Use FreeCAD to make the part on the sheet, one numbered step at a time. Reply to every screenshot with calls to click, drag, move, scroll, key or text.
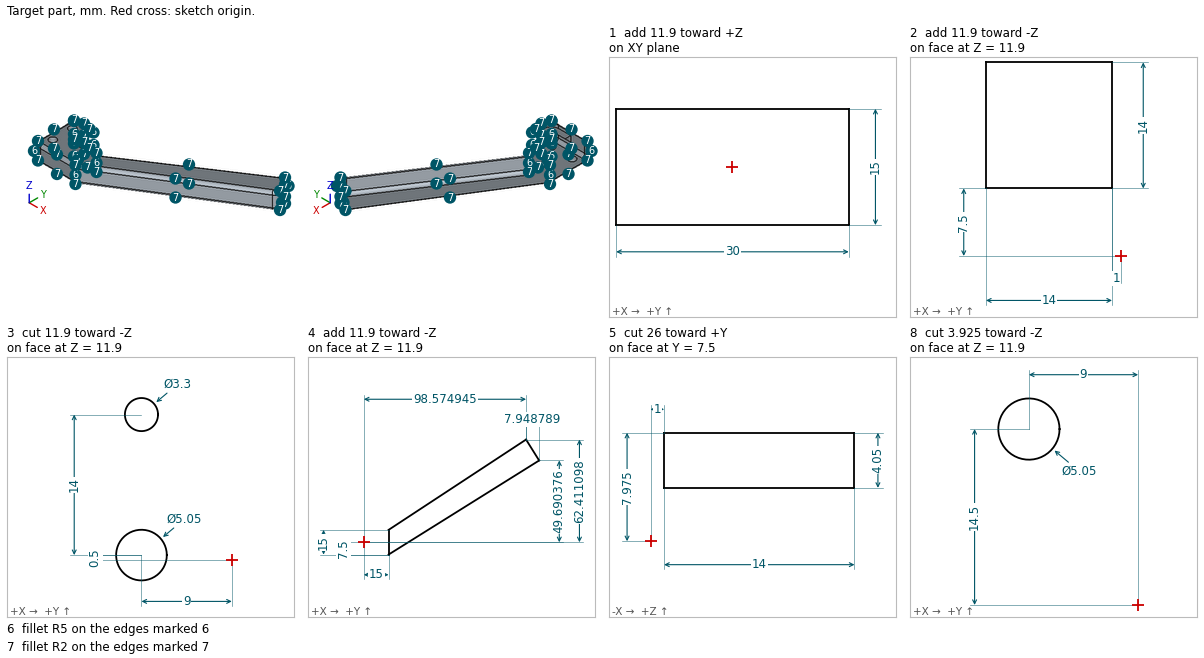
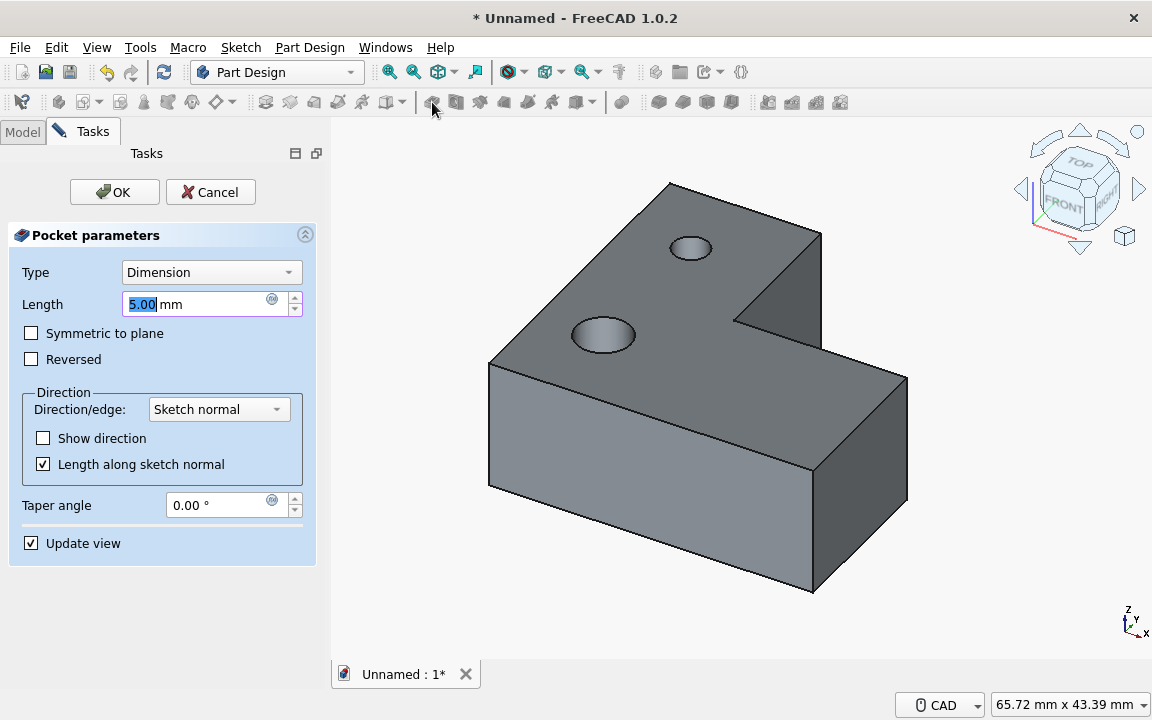
text(11.9)
key(Tab)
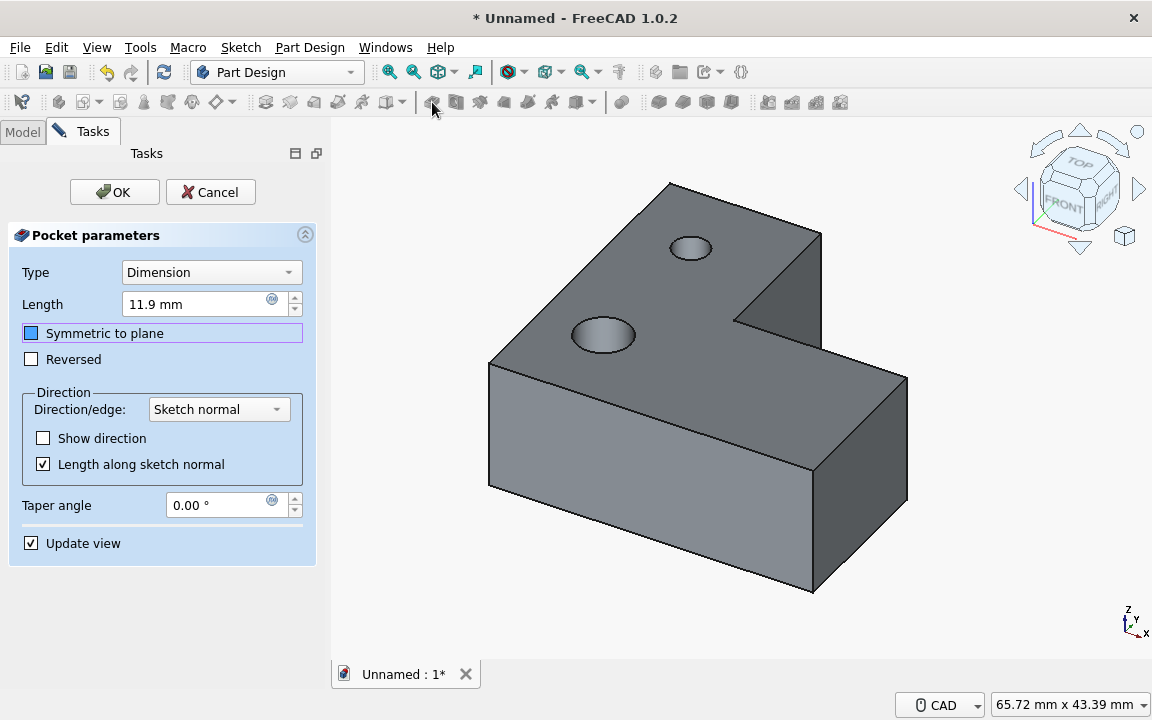
click(115, 192)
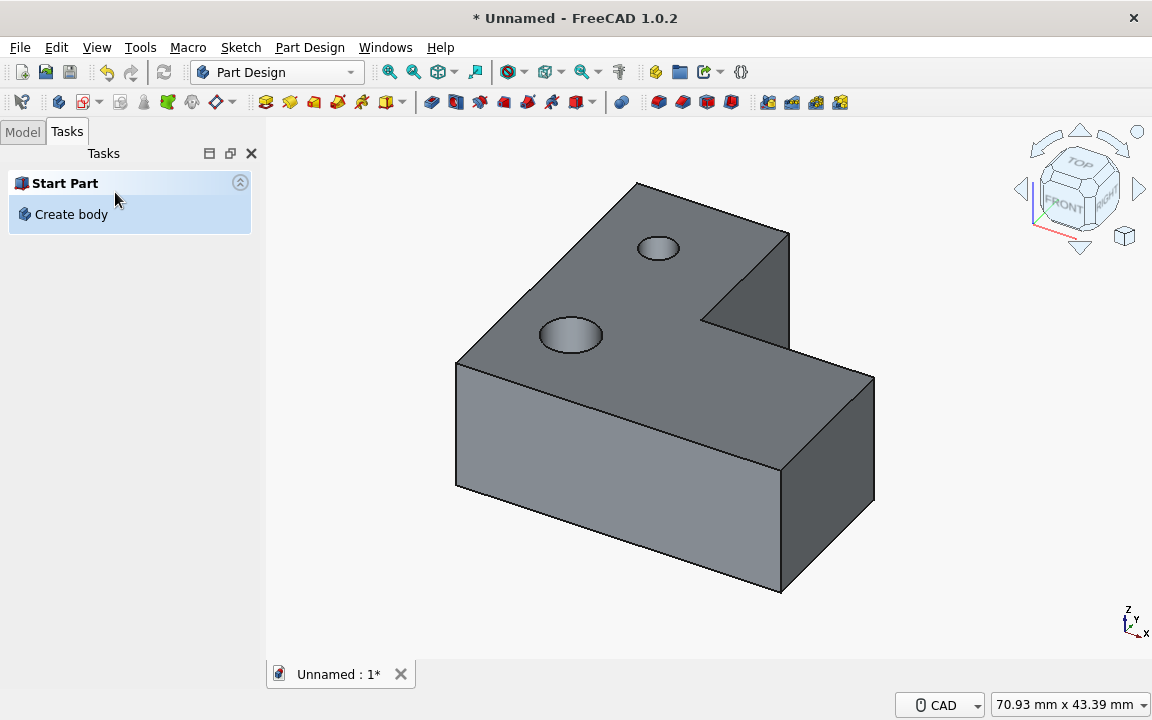
click(750, 408)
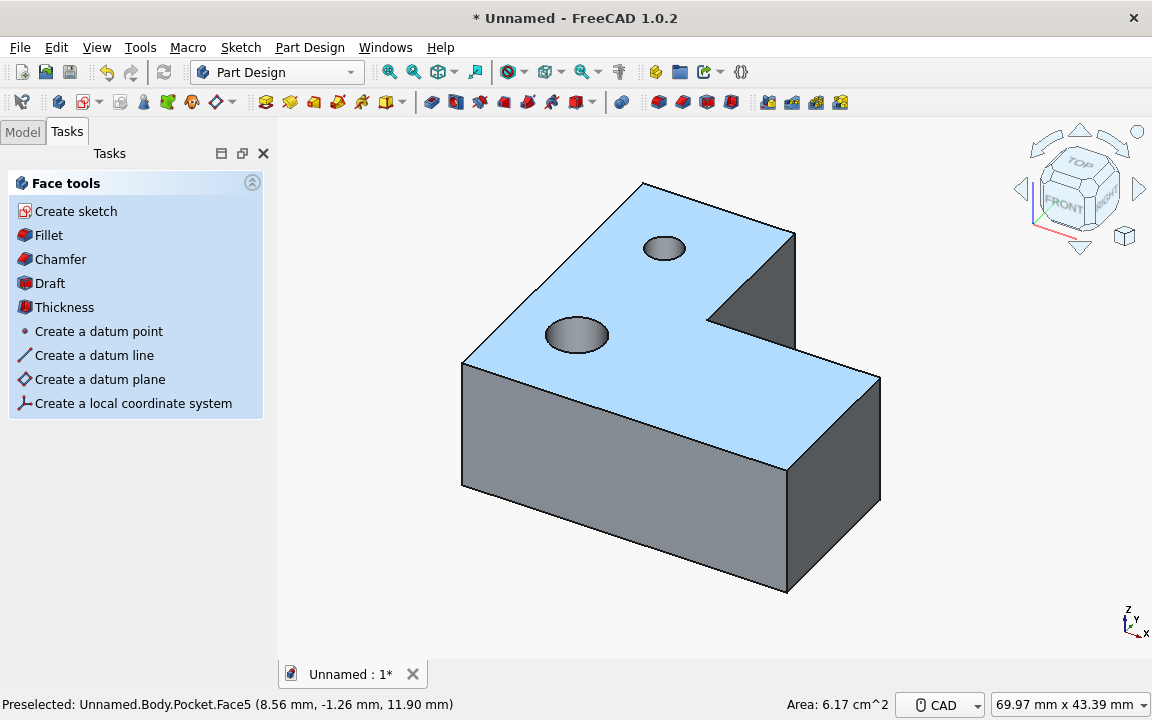
click(84, 102)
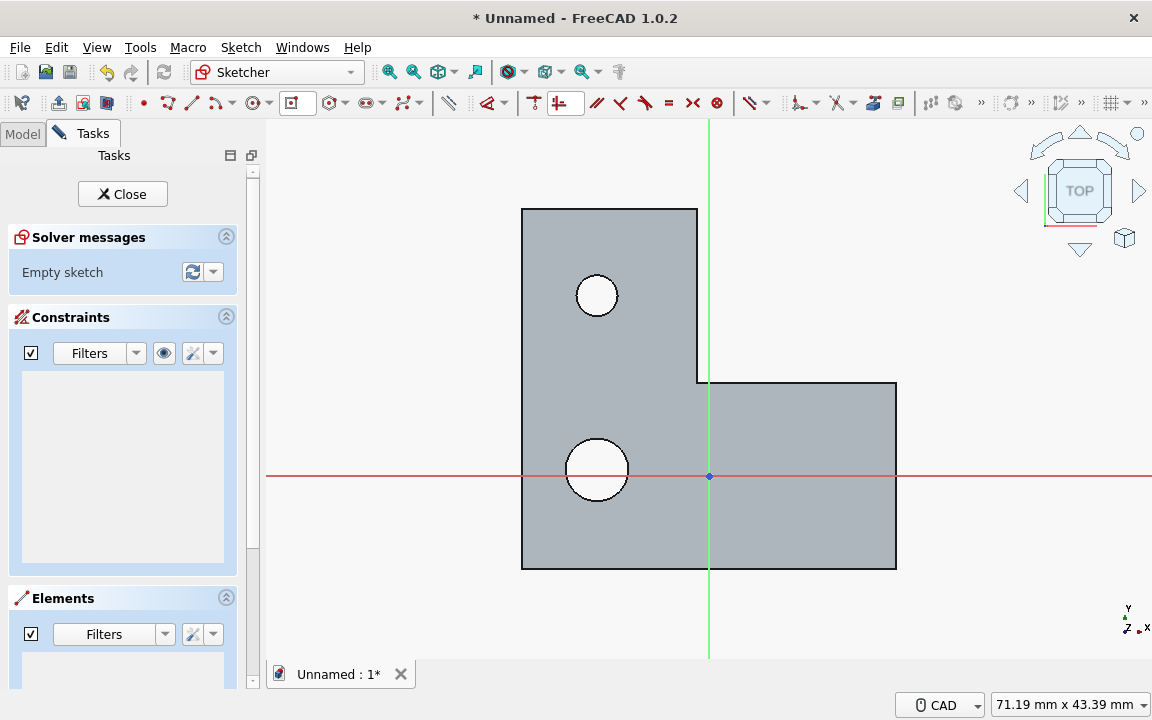
scroll(294, 537, down, 5)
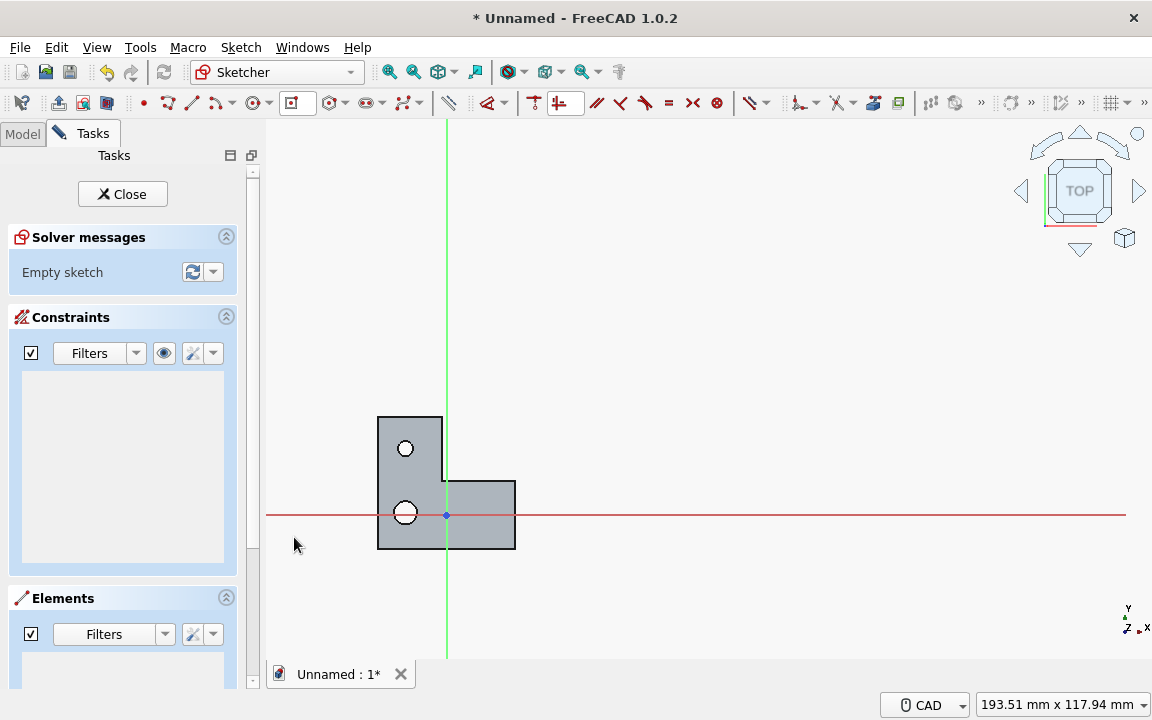
click(168, 104)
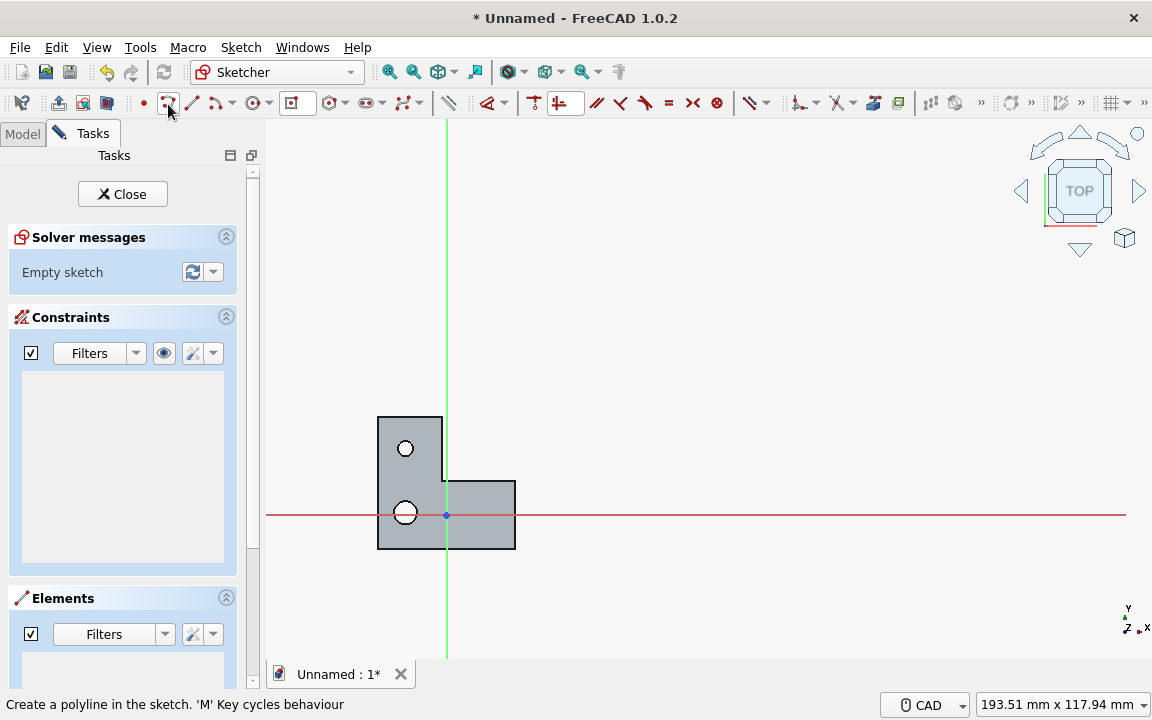
click(515, 549)
click(934, 288)
click(898, 229)
click(515, 481)
click(515, 550)
key(Escape)
key(Escape)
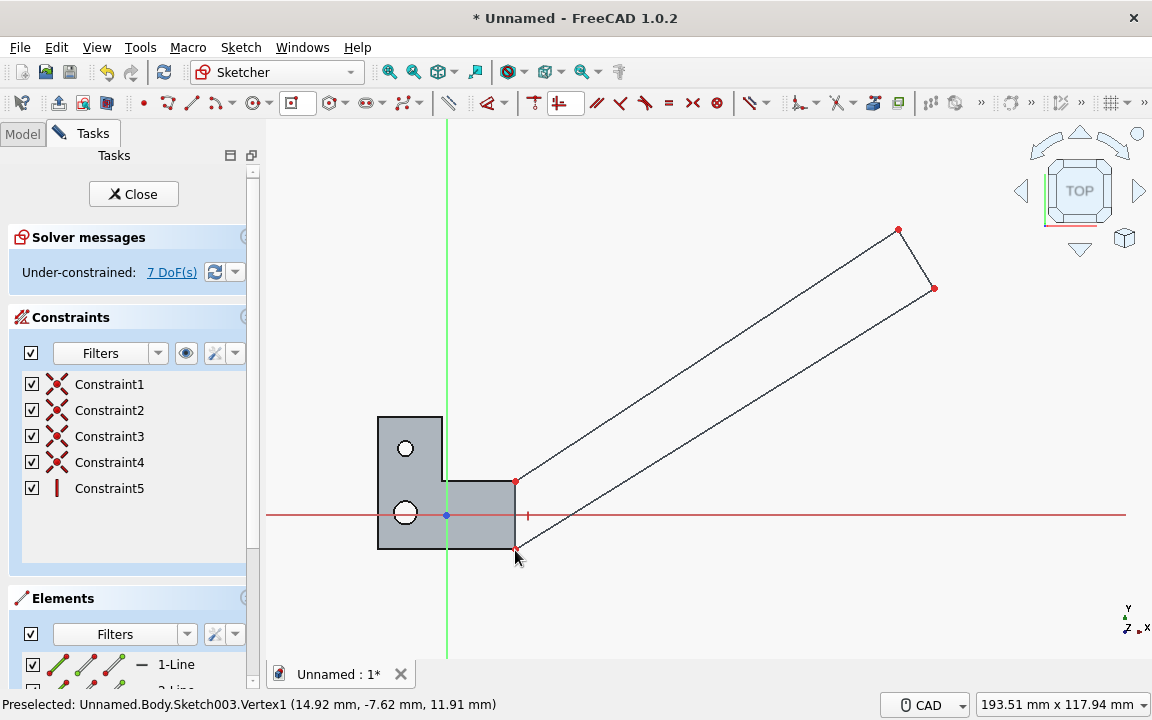
click(488, 104)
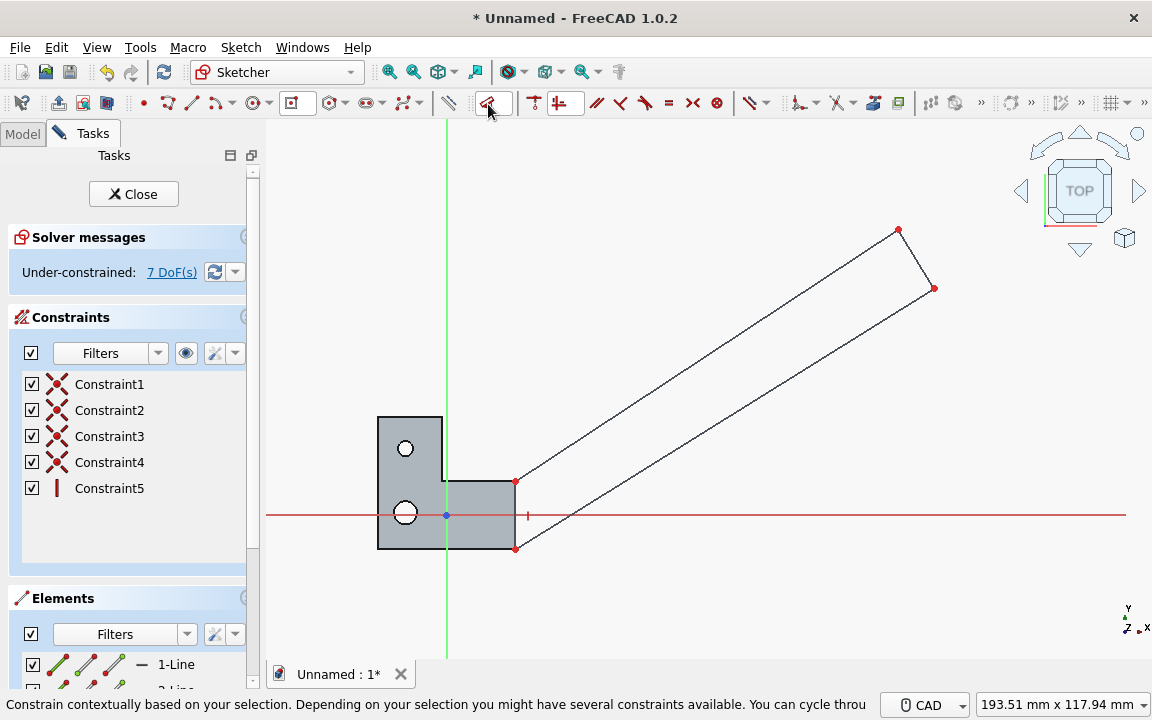
click(515, 502)
click(481, 500)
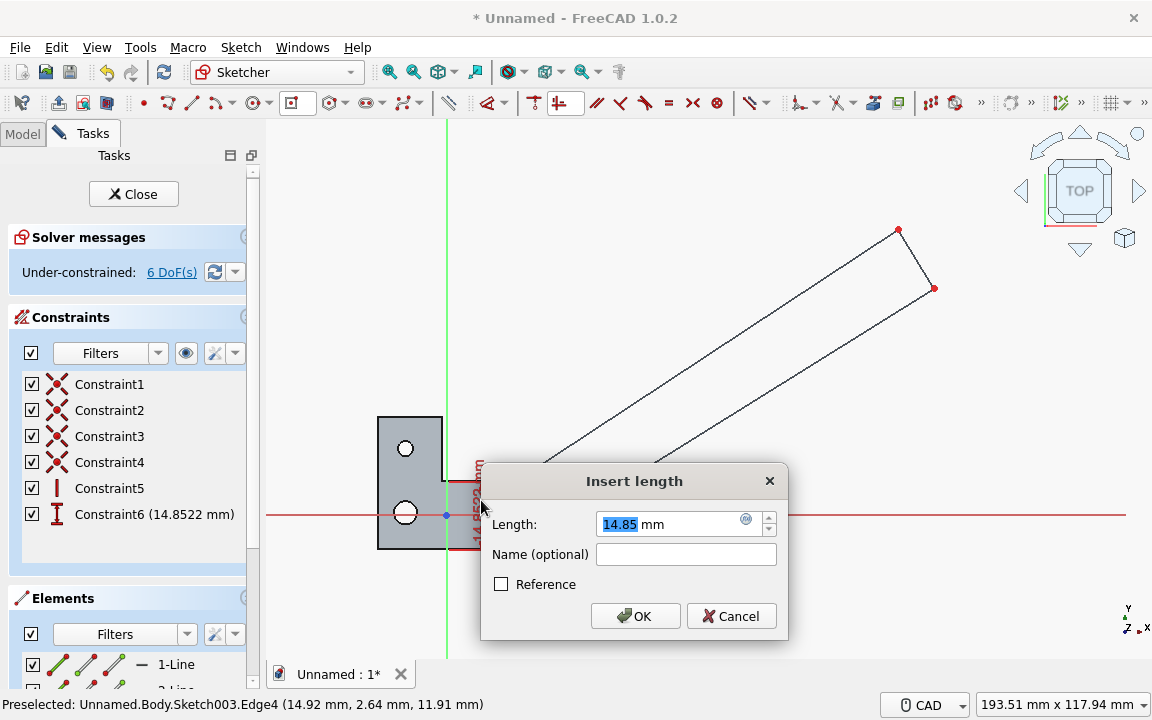
text(15)
key(Return)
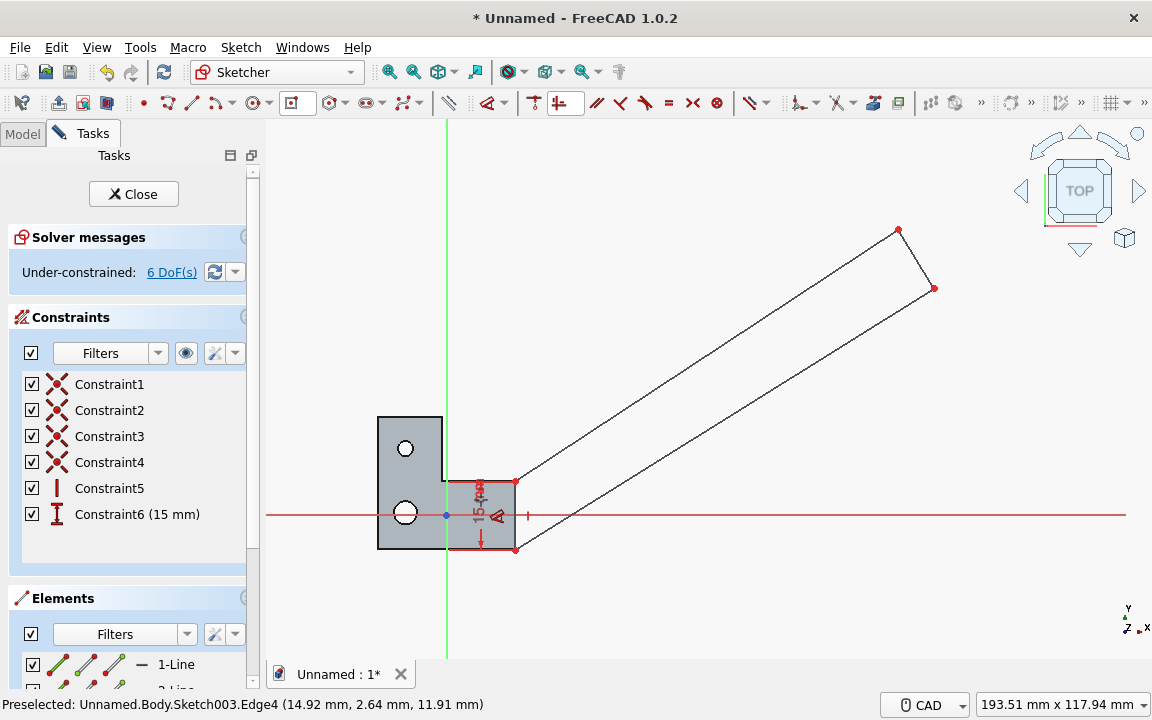
click(515, 550)
click(481, 584)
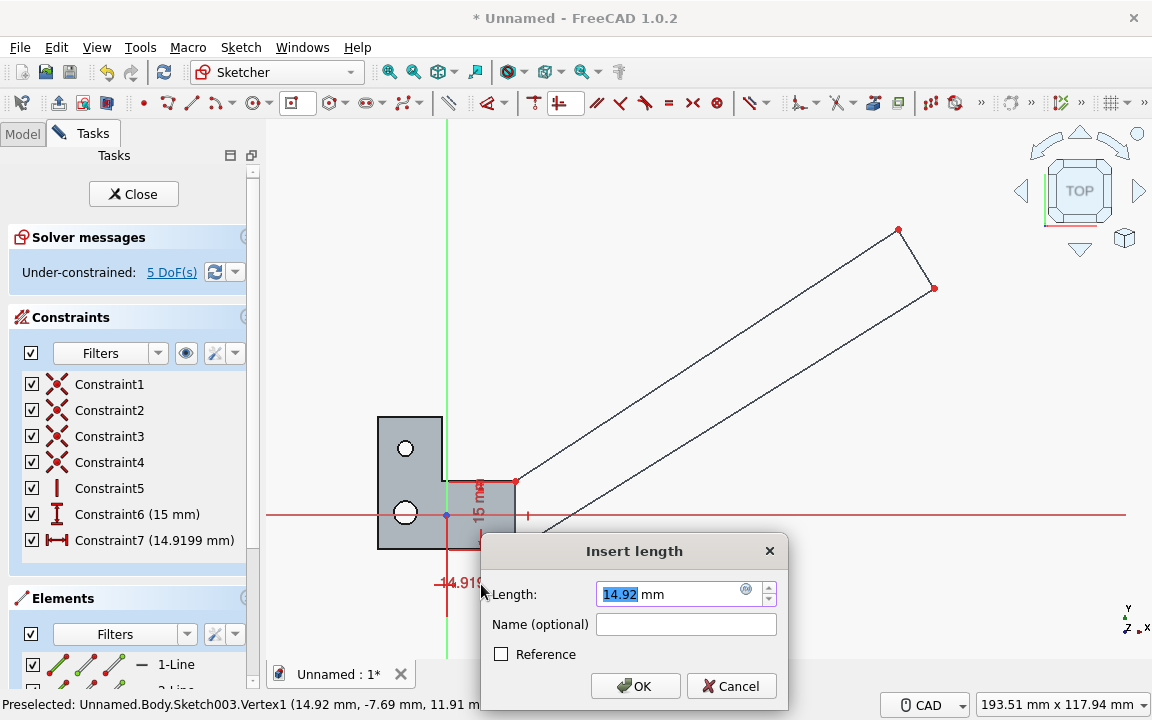
text(15)
key(Return)